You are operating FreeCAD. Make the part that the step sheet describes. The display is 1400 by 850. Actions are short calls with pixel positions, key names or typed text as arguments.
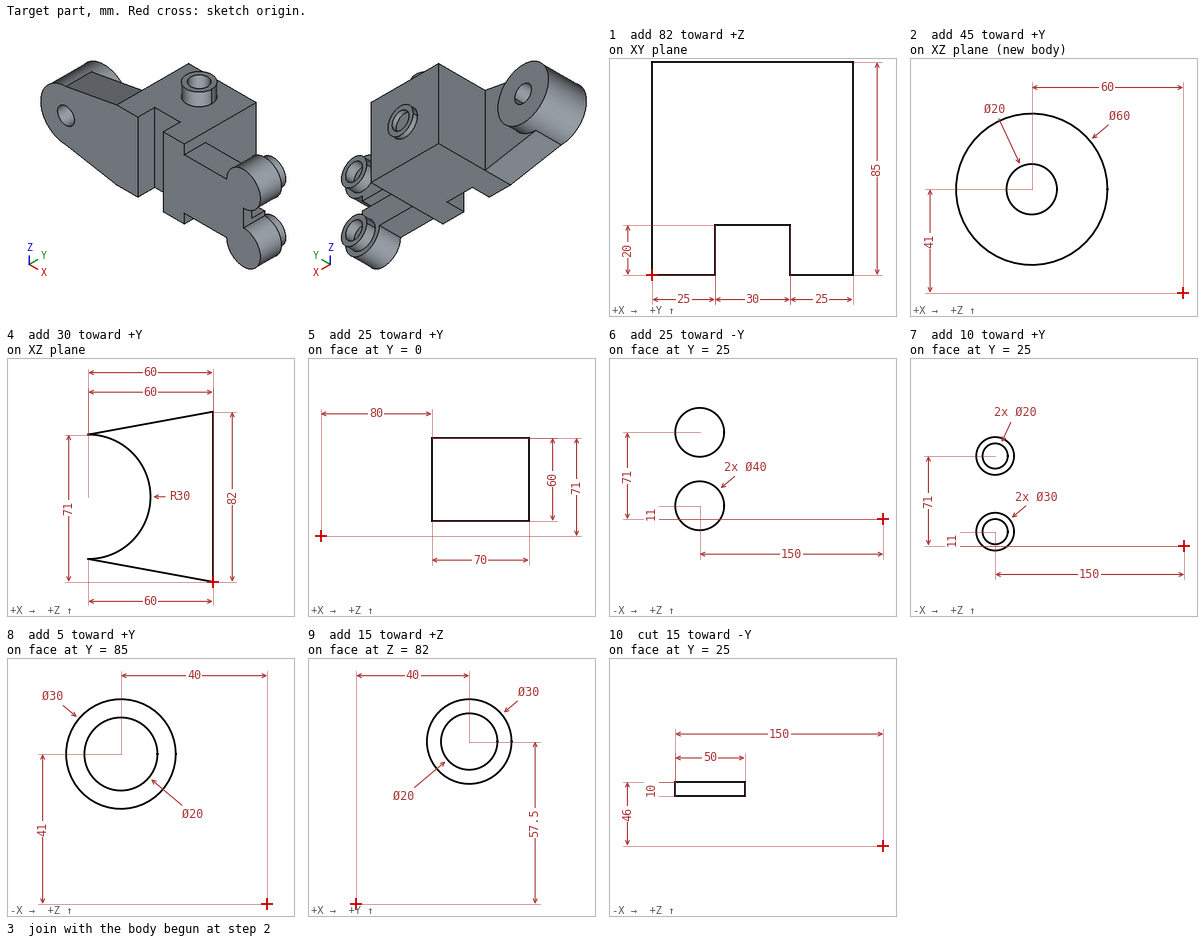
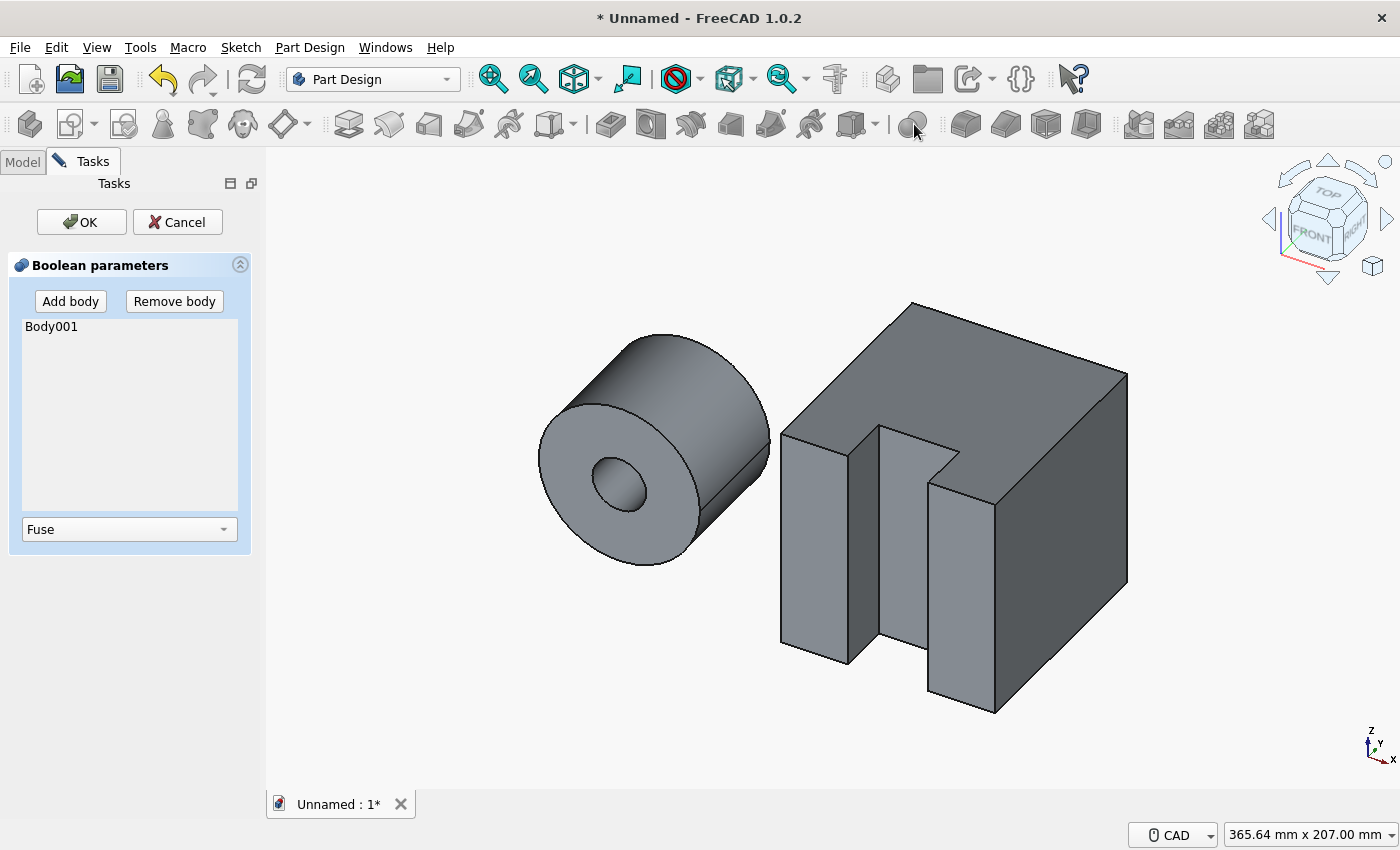
click(82, 222)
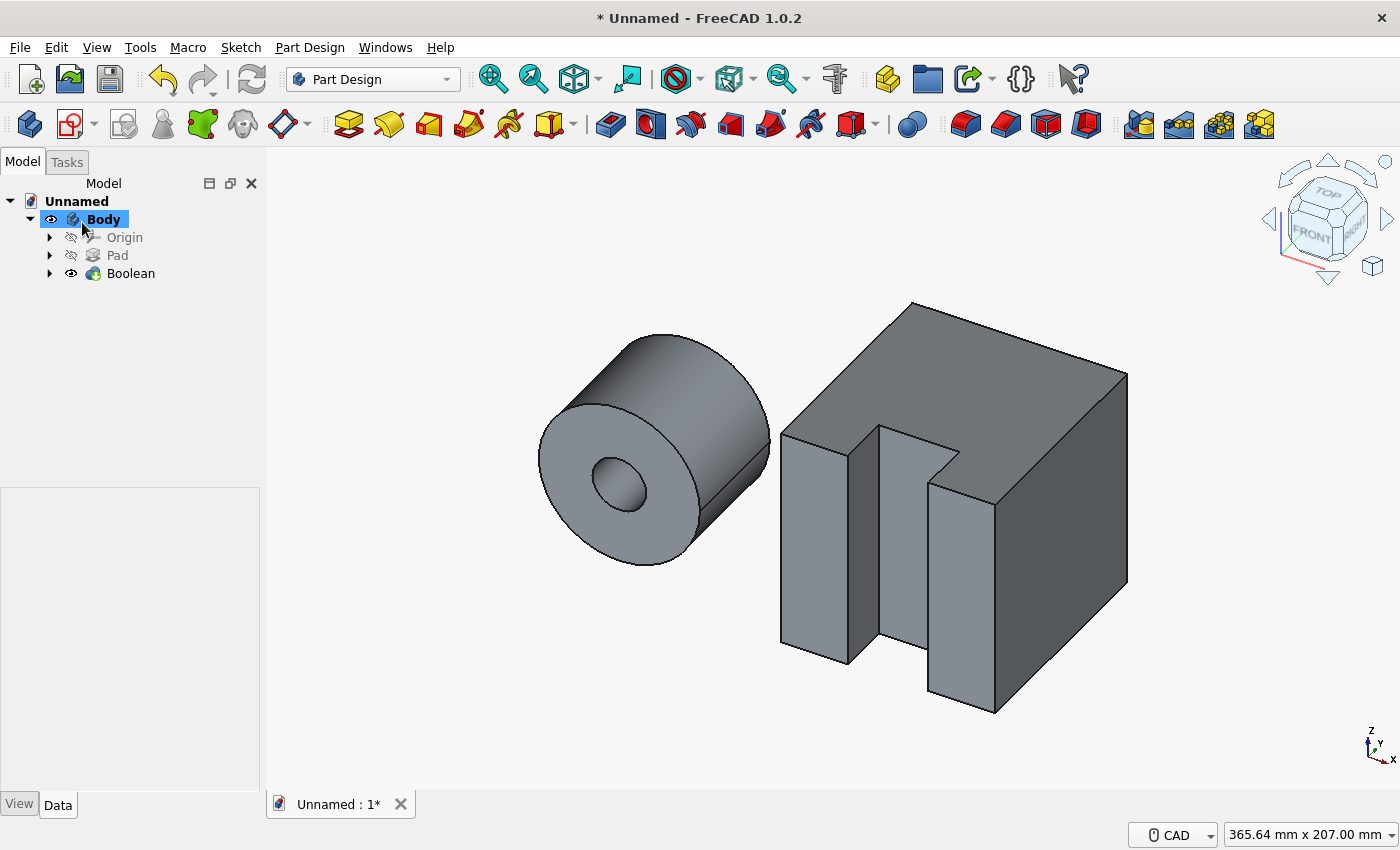
click(70, 124)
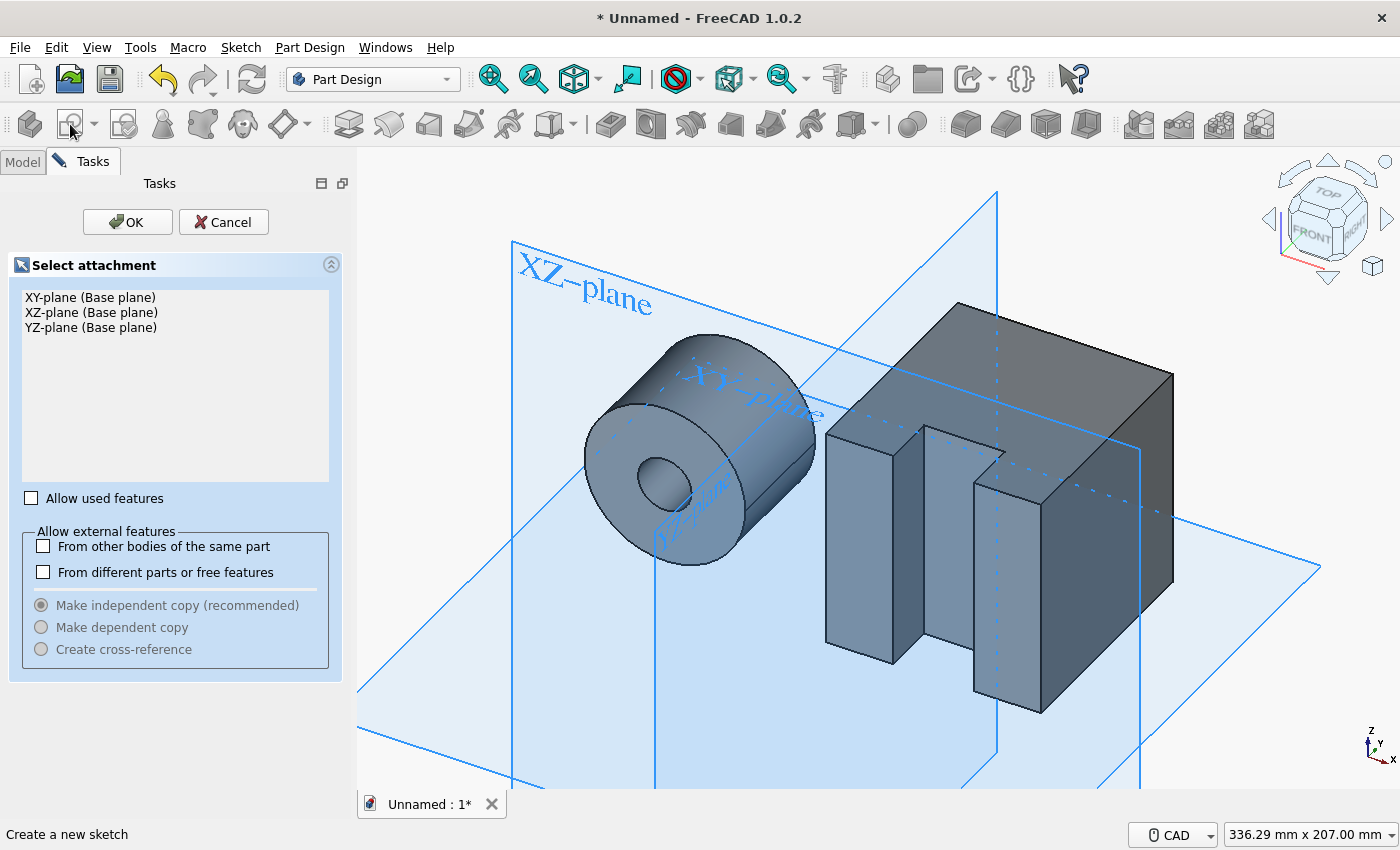
click(82, 312)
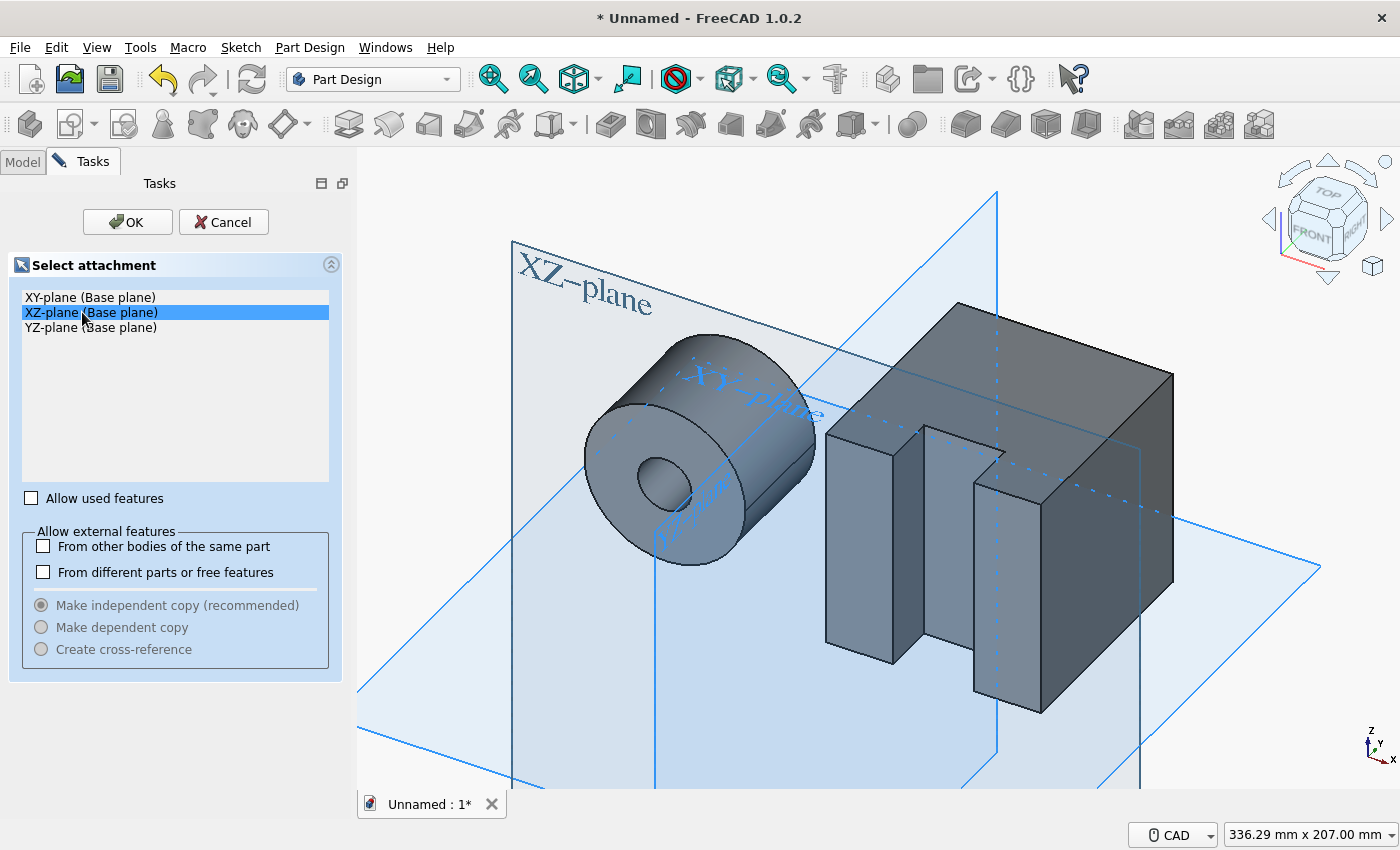
click(128, 222)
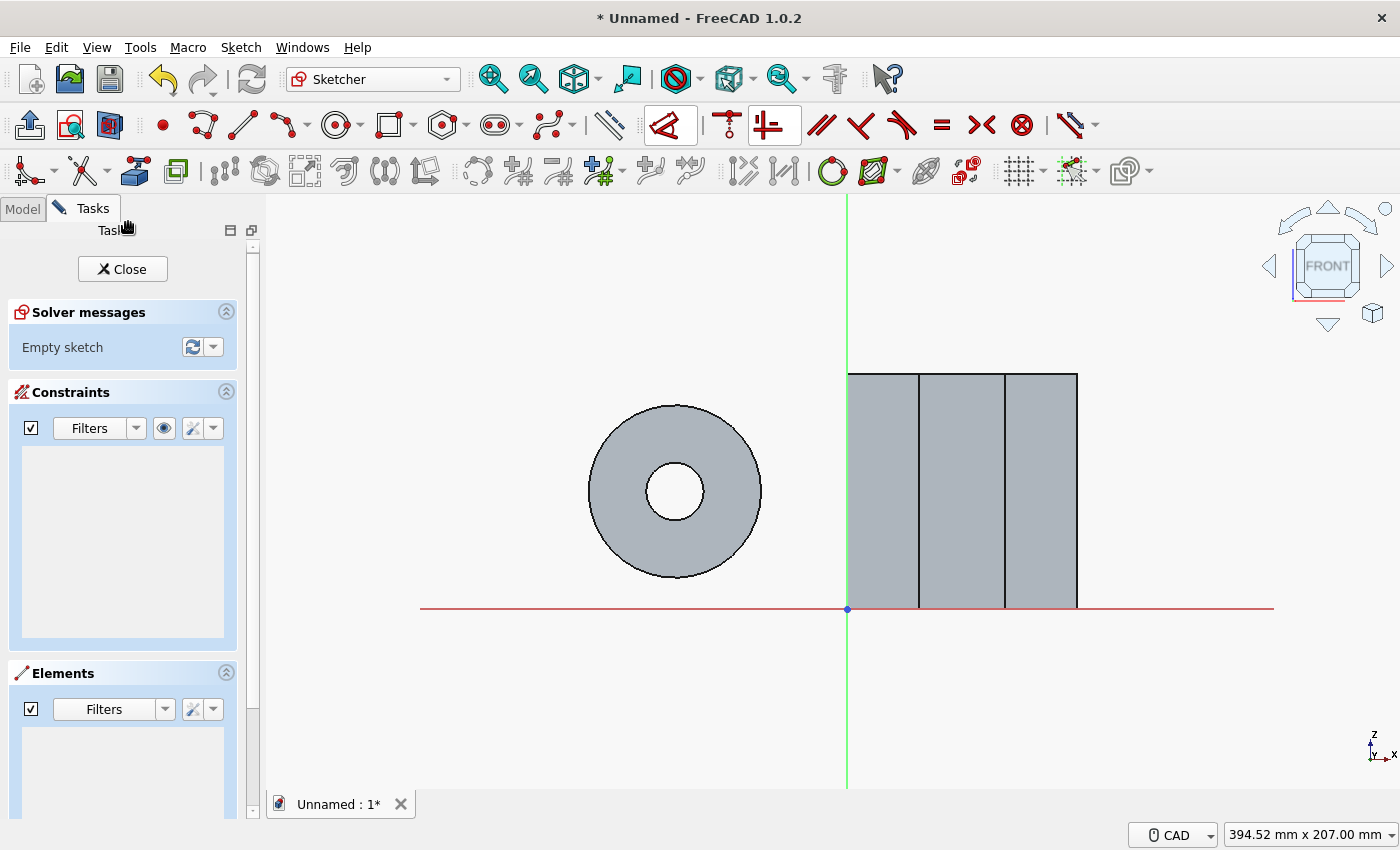
scroll(754, 492, up, 2)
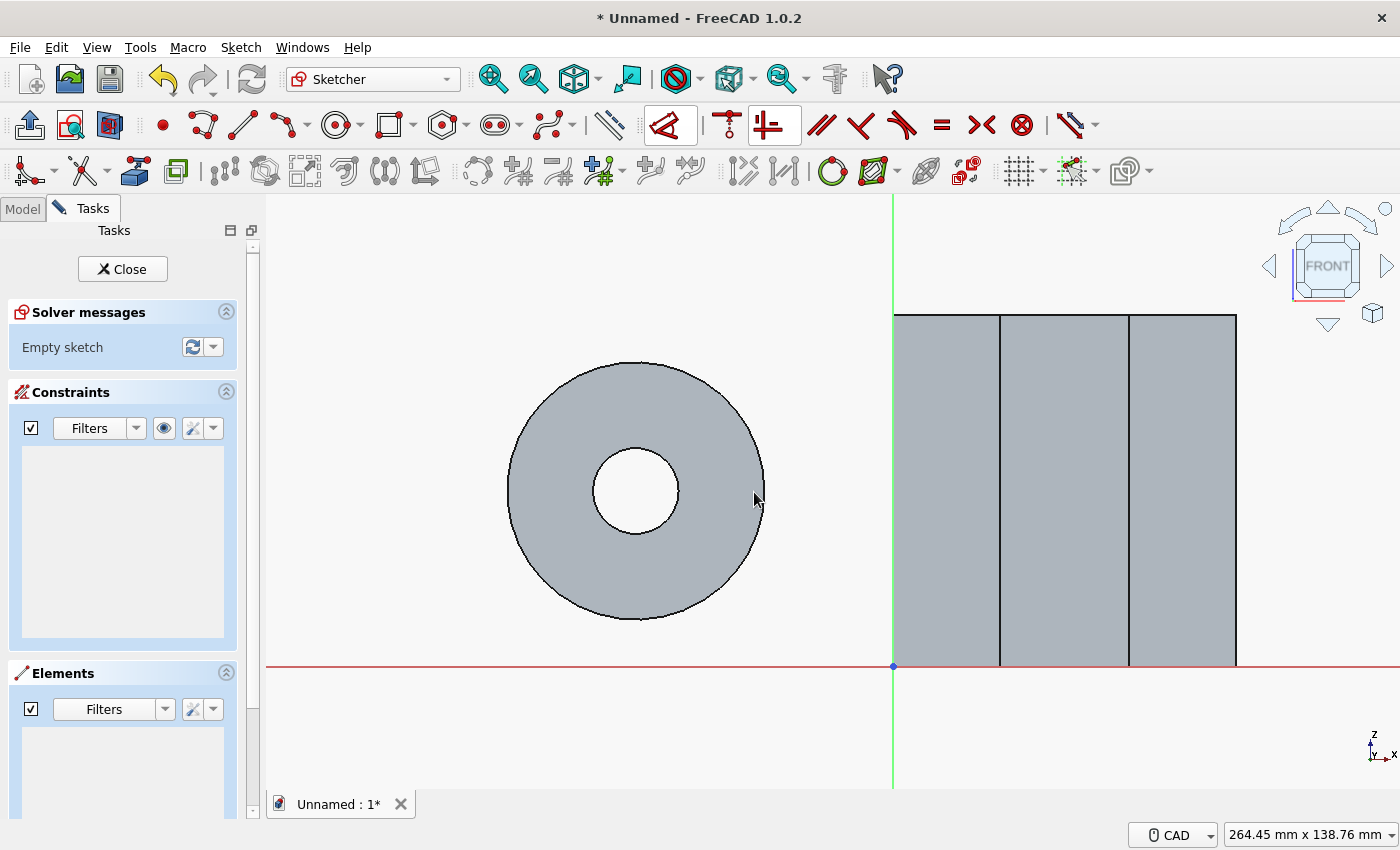
click(204, 126)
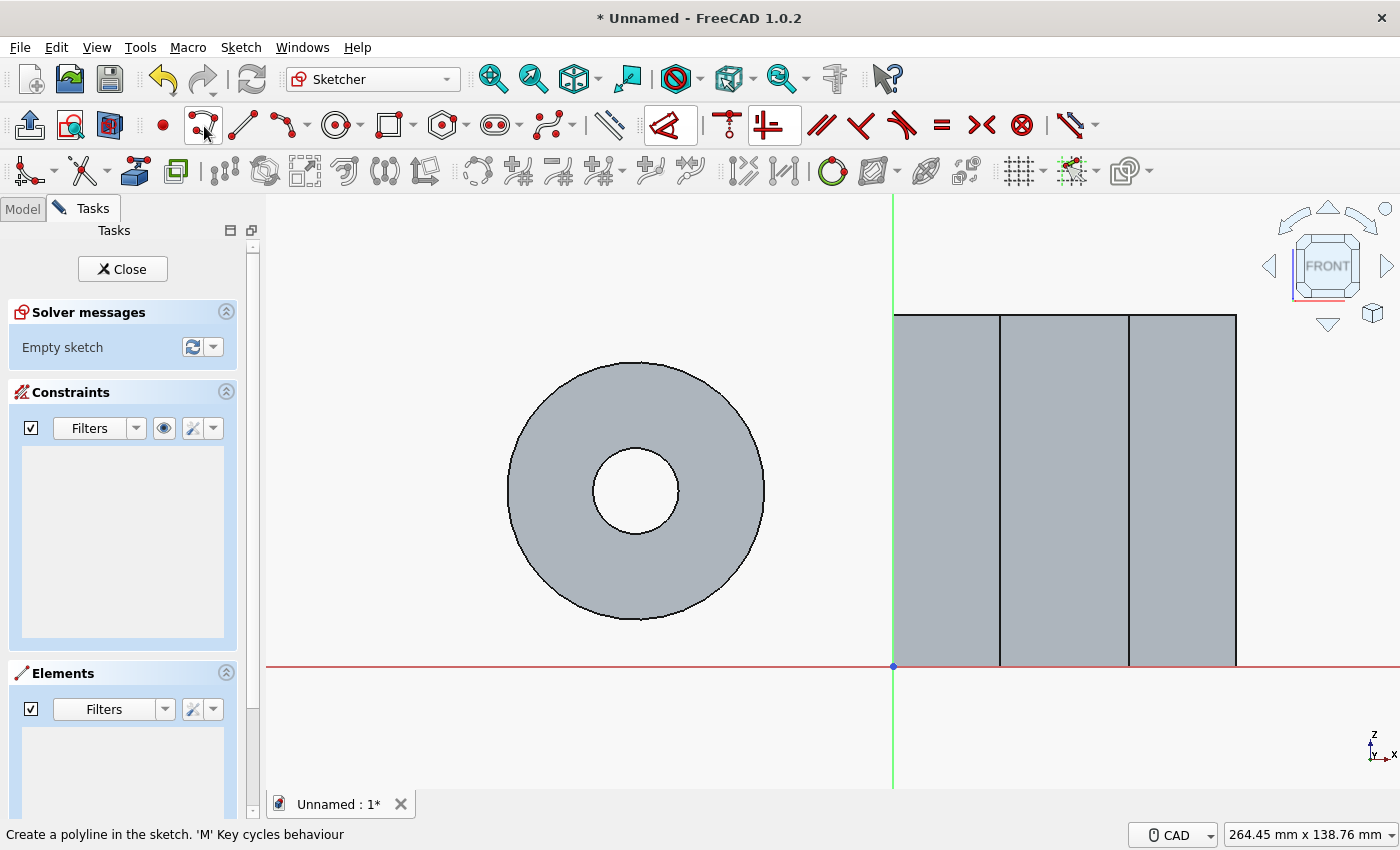
click(636, 362)
click(893, 315)
click(893, 667)
click(636, 620)
right_click(636, 620)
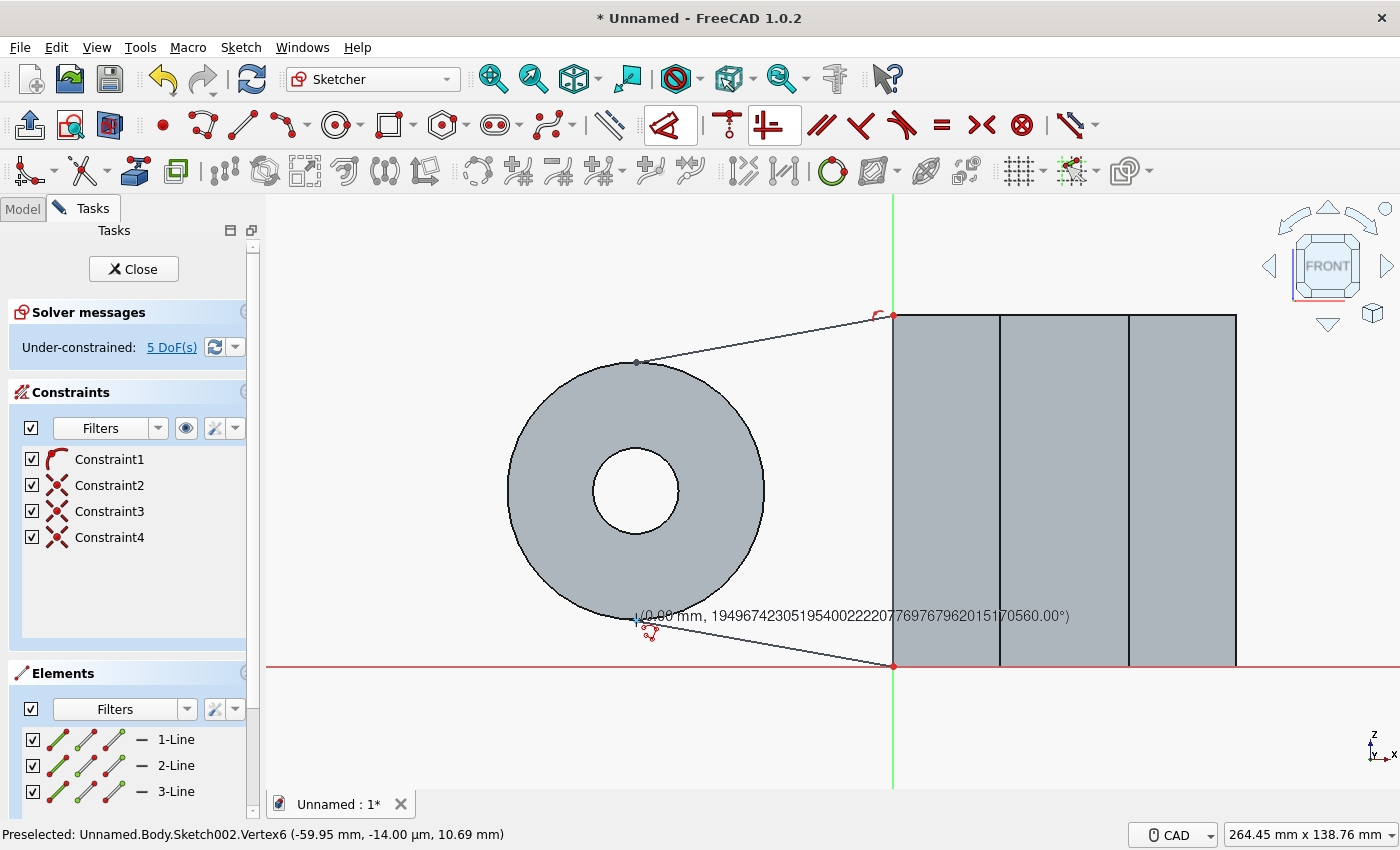
click(284, 126)